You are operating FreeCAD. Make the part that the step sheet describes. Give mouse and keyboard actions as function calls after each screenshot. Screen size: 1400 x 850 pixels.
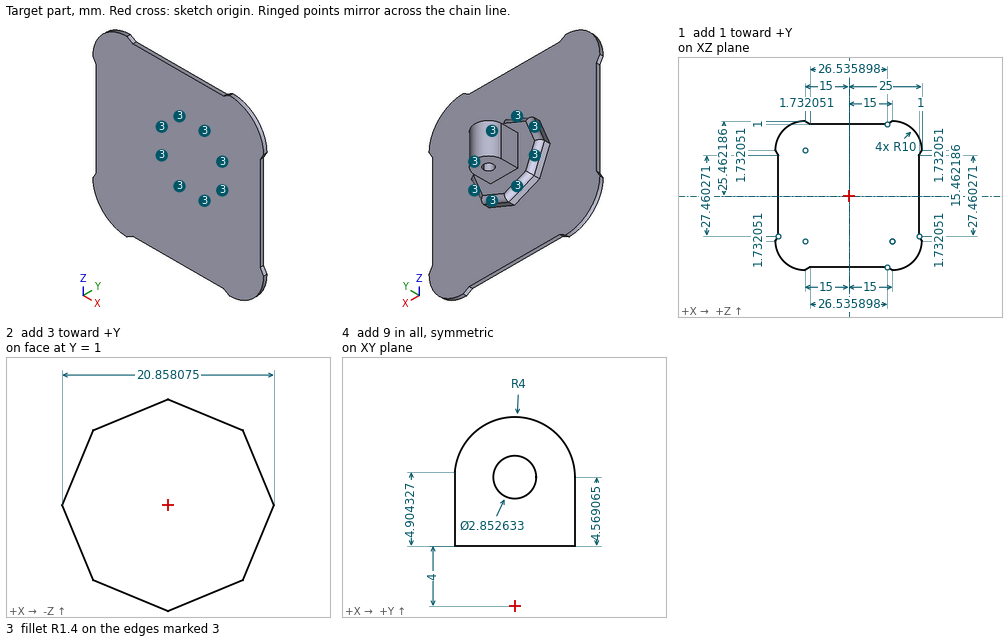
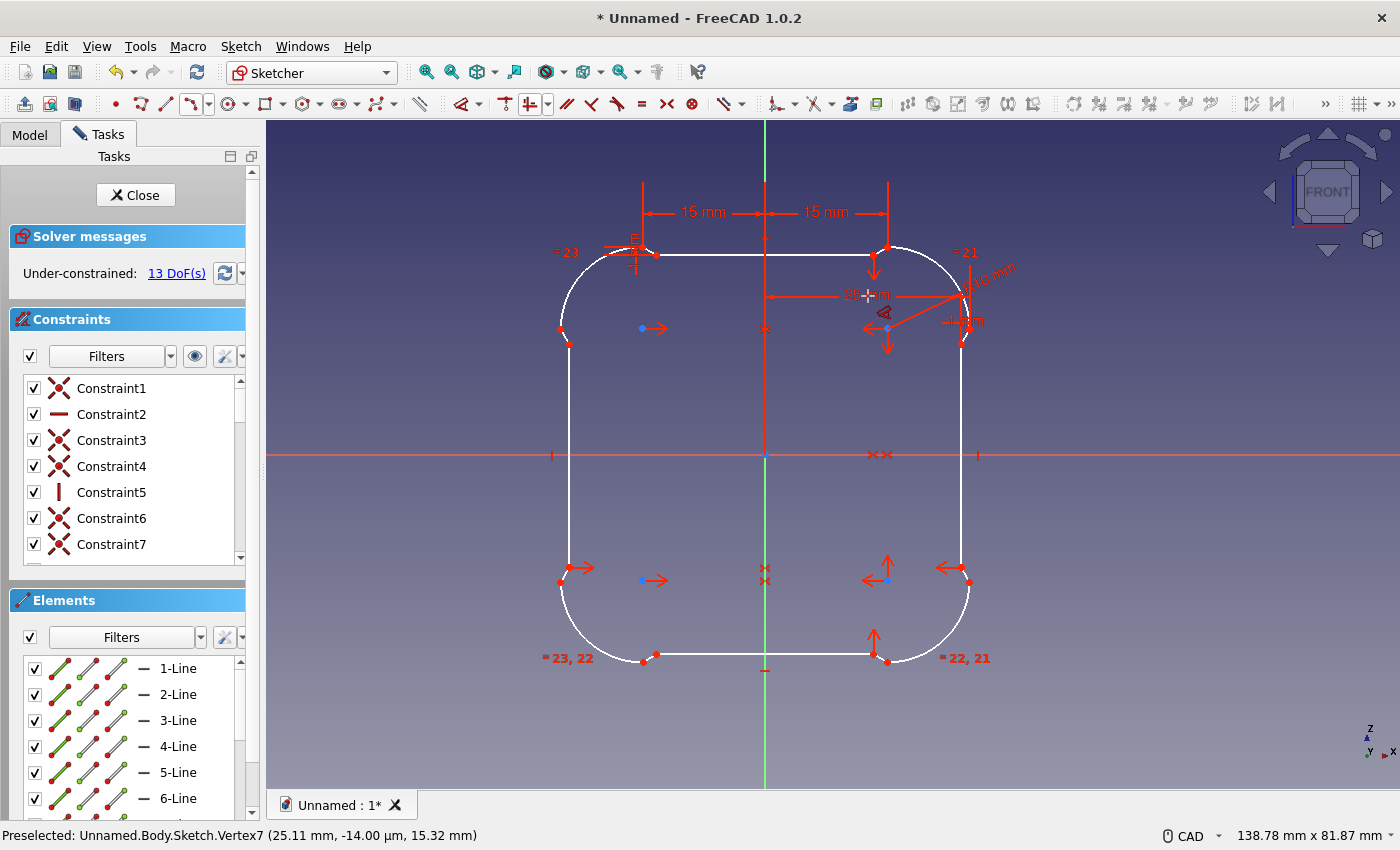
click(887, 662)
click(826, 696)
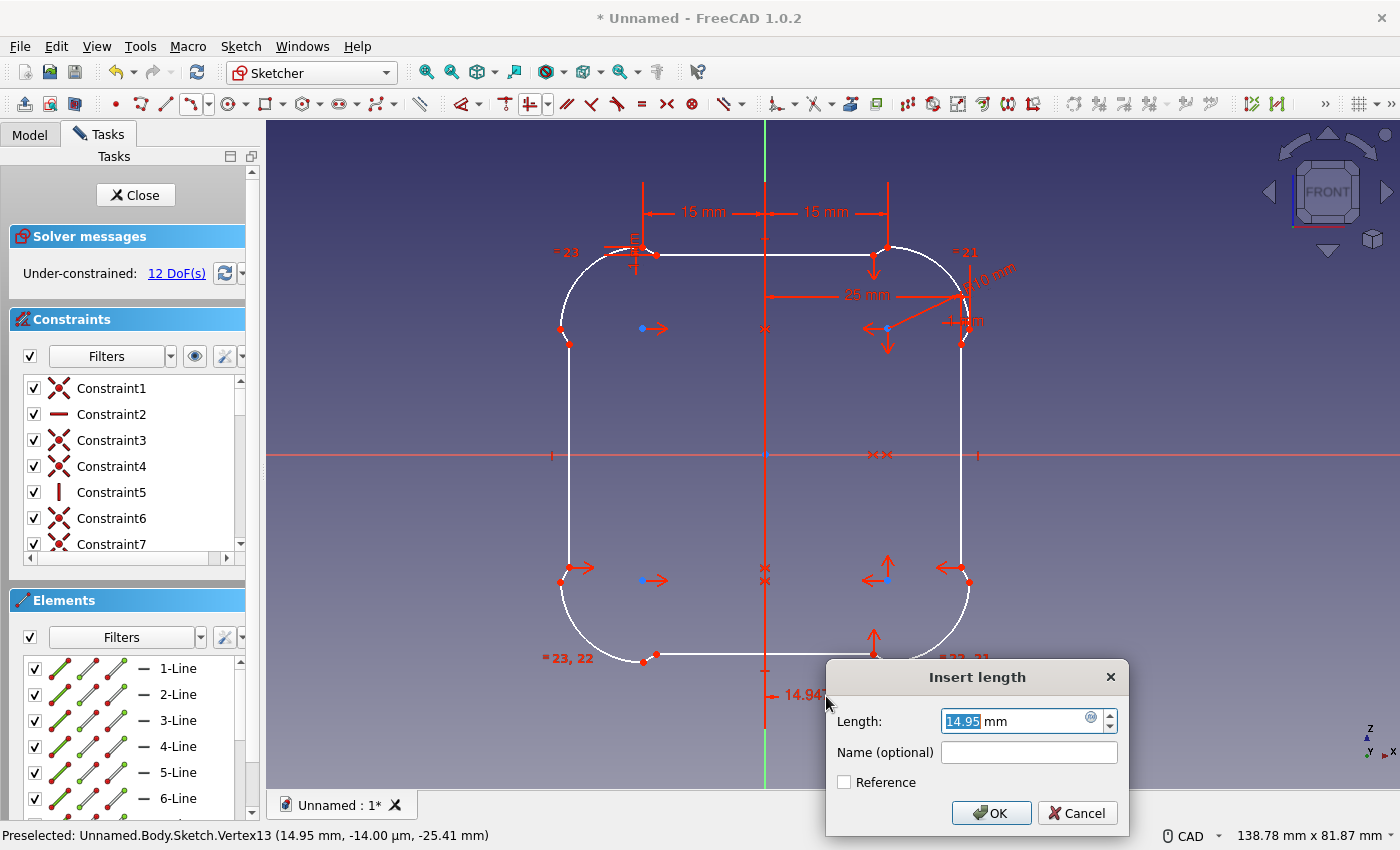
text(15)
key(Return)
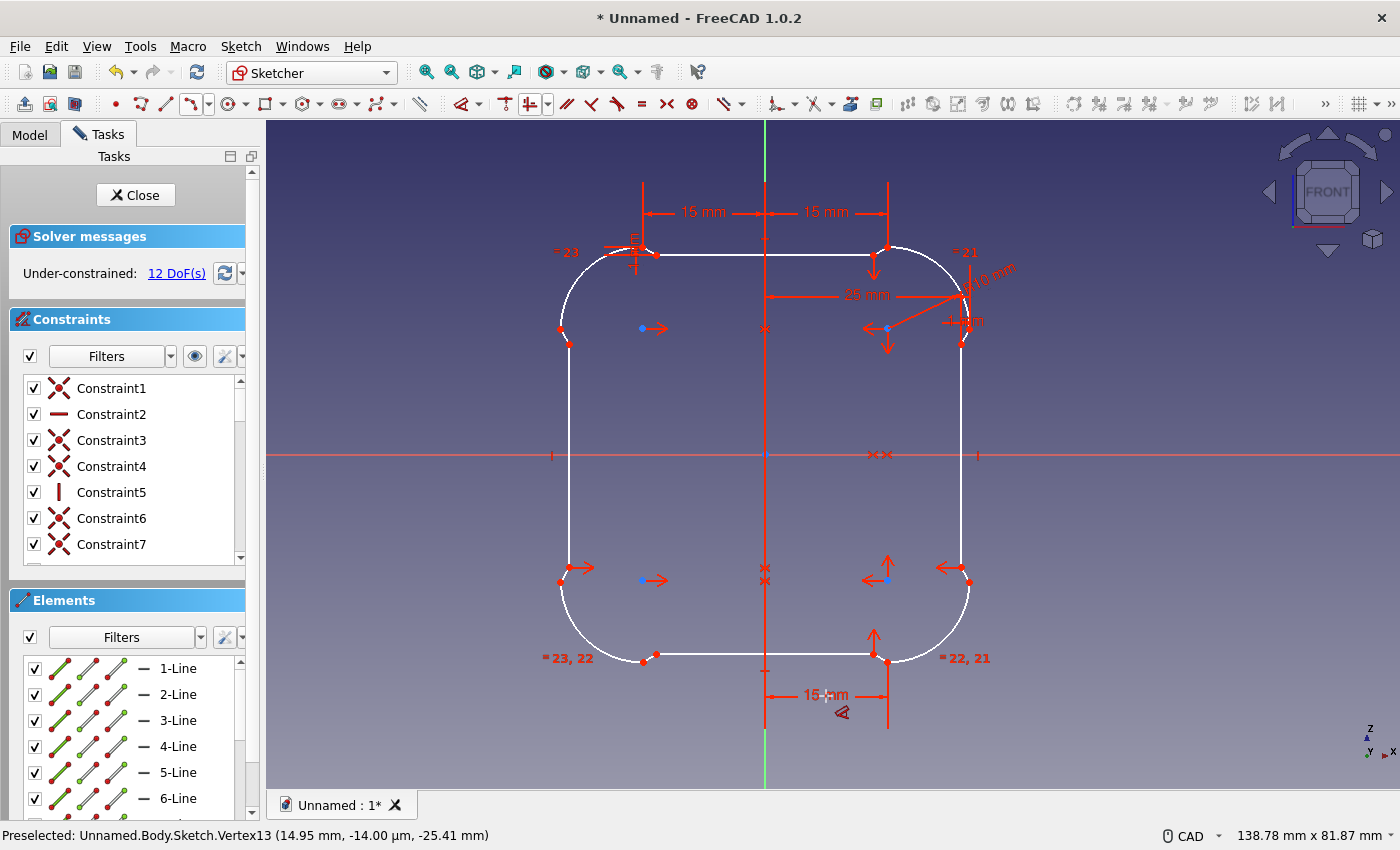
click(643, 662)
click(704, 696)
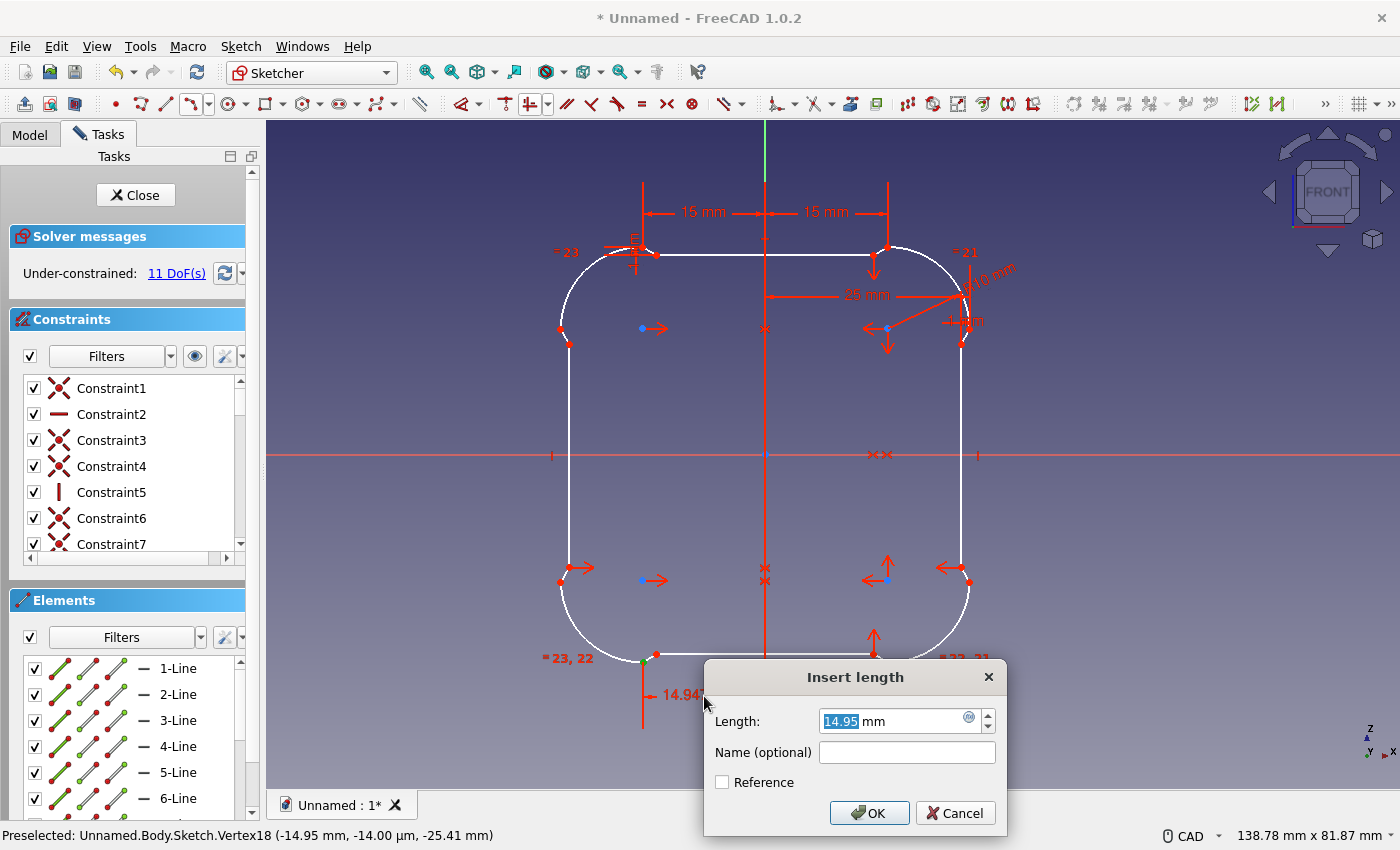
text(15)
key(Return)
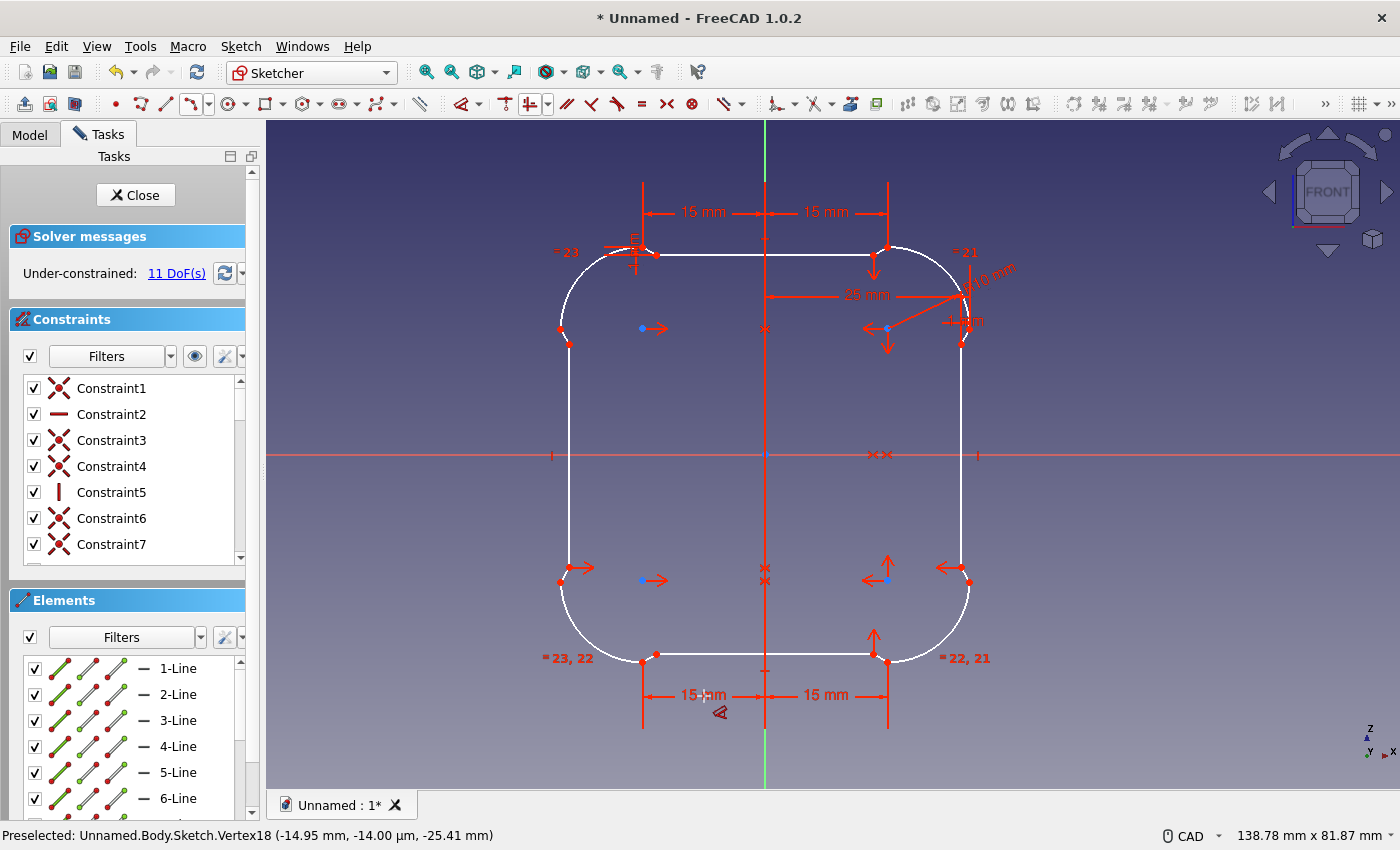
click(722, 255)
click(715, 289)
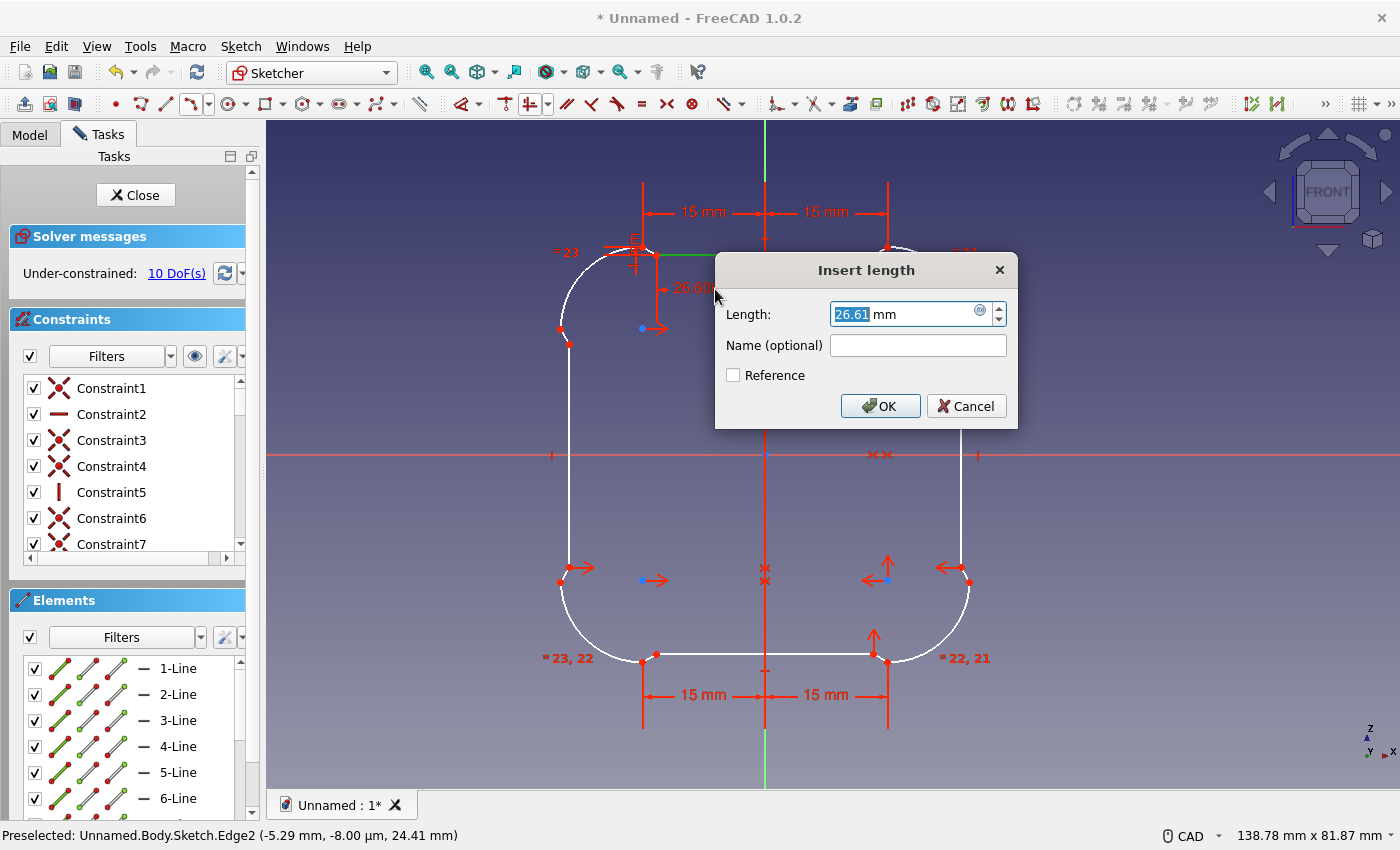
text(26.535898)
key(Return)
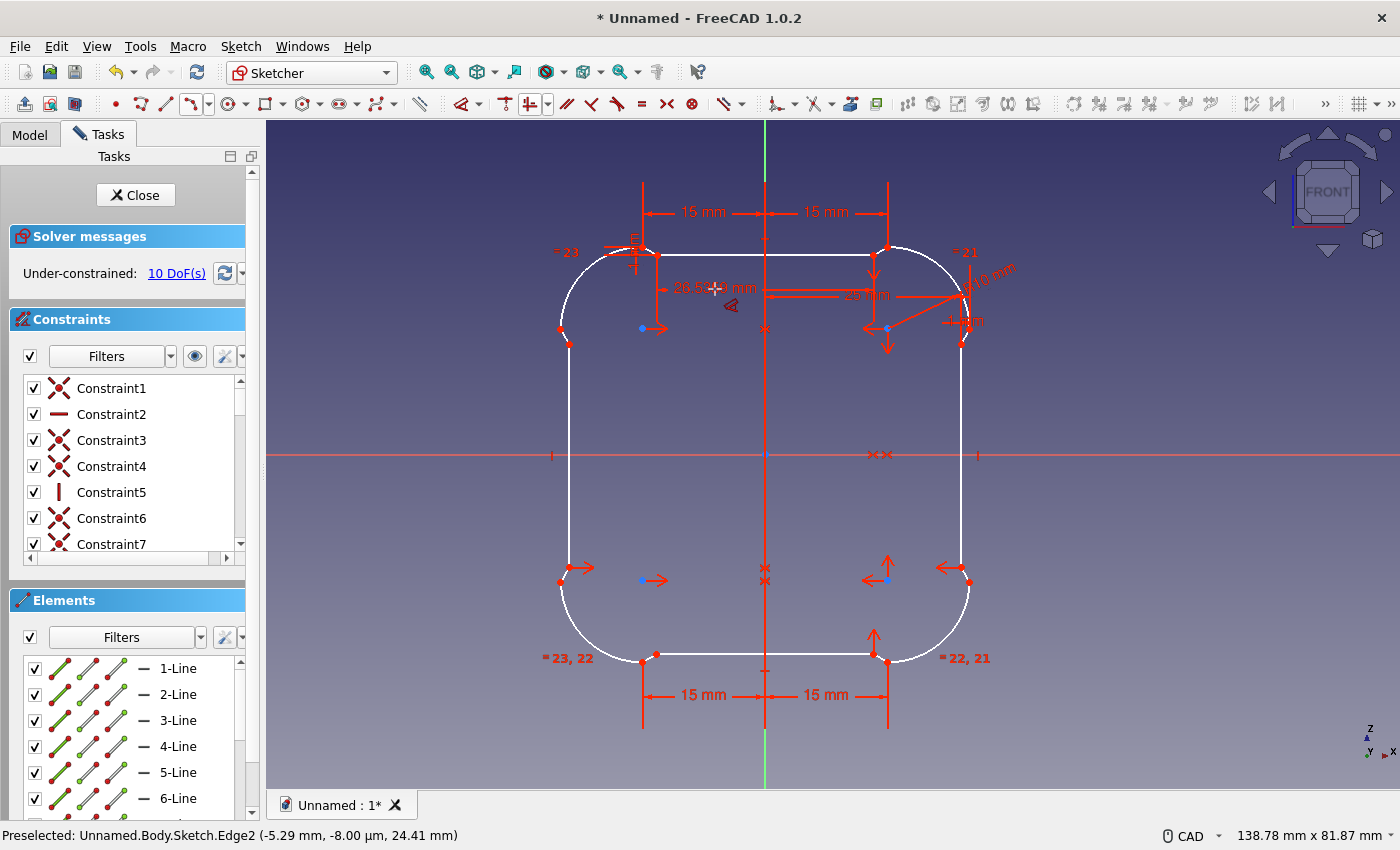
click(961, 411)
click(995, 405)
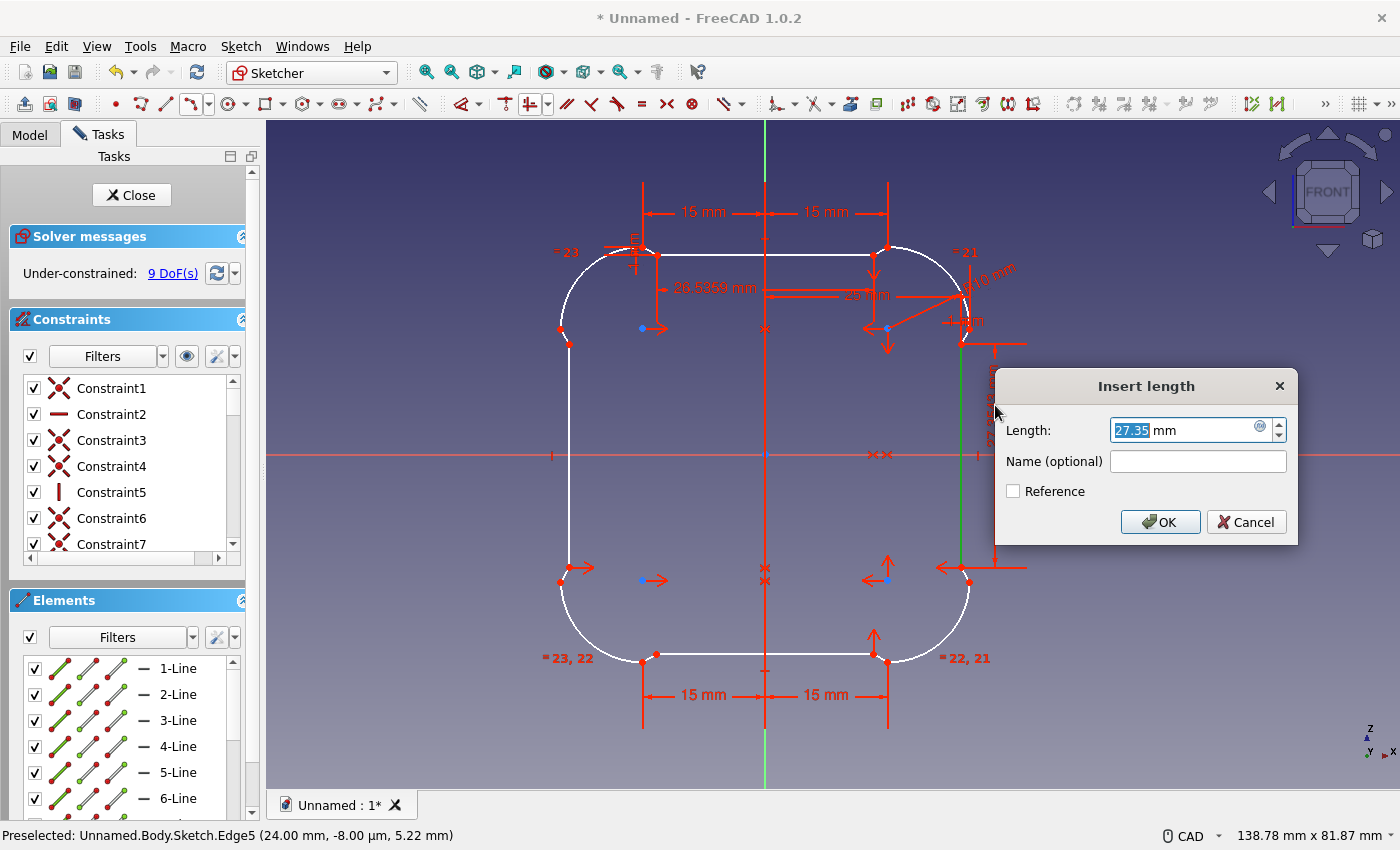
text(27.460271)
key(Return)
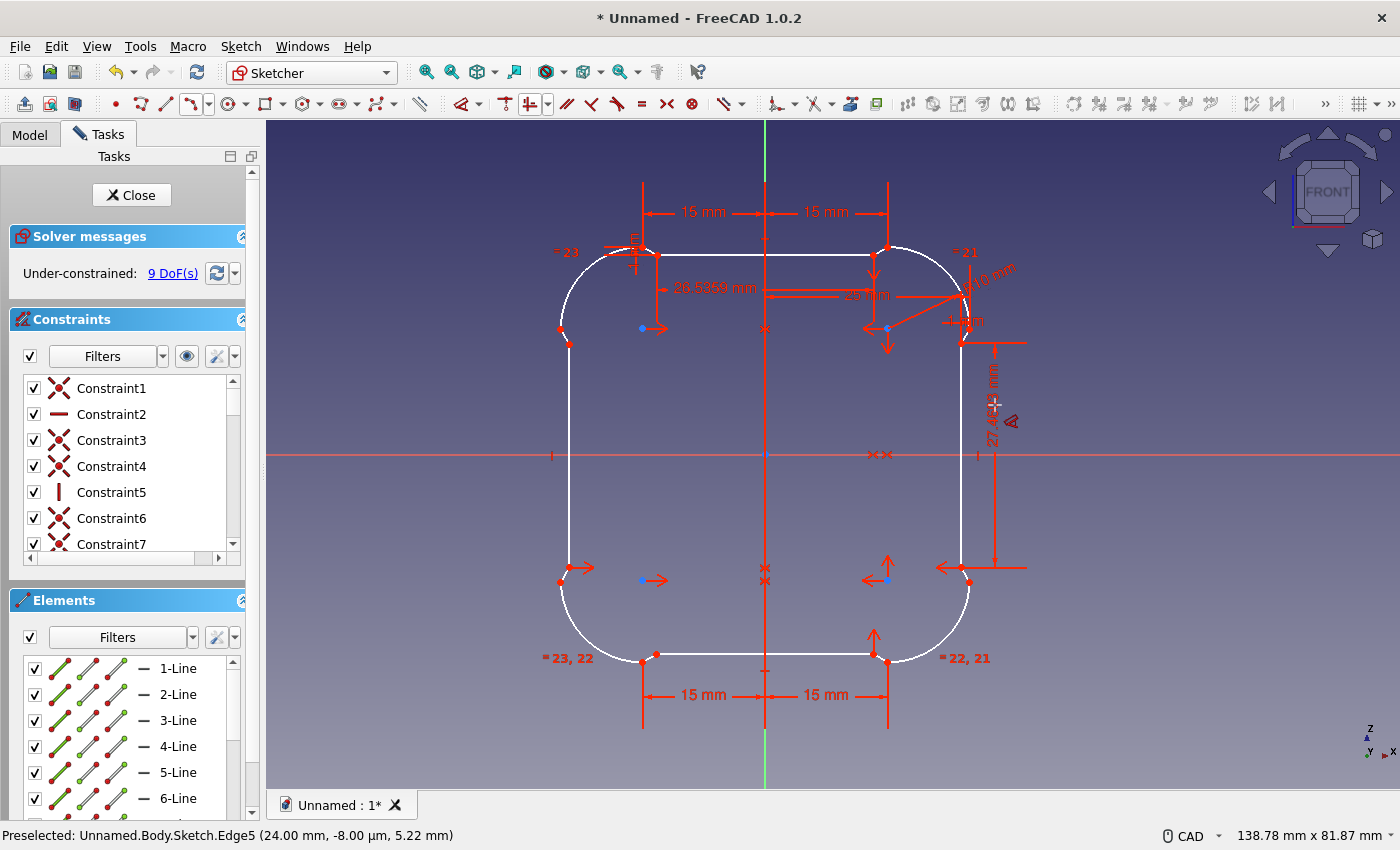
click(809, 654)
click(715, 620)